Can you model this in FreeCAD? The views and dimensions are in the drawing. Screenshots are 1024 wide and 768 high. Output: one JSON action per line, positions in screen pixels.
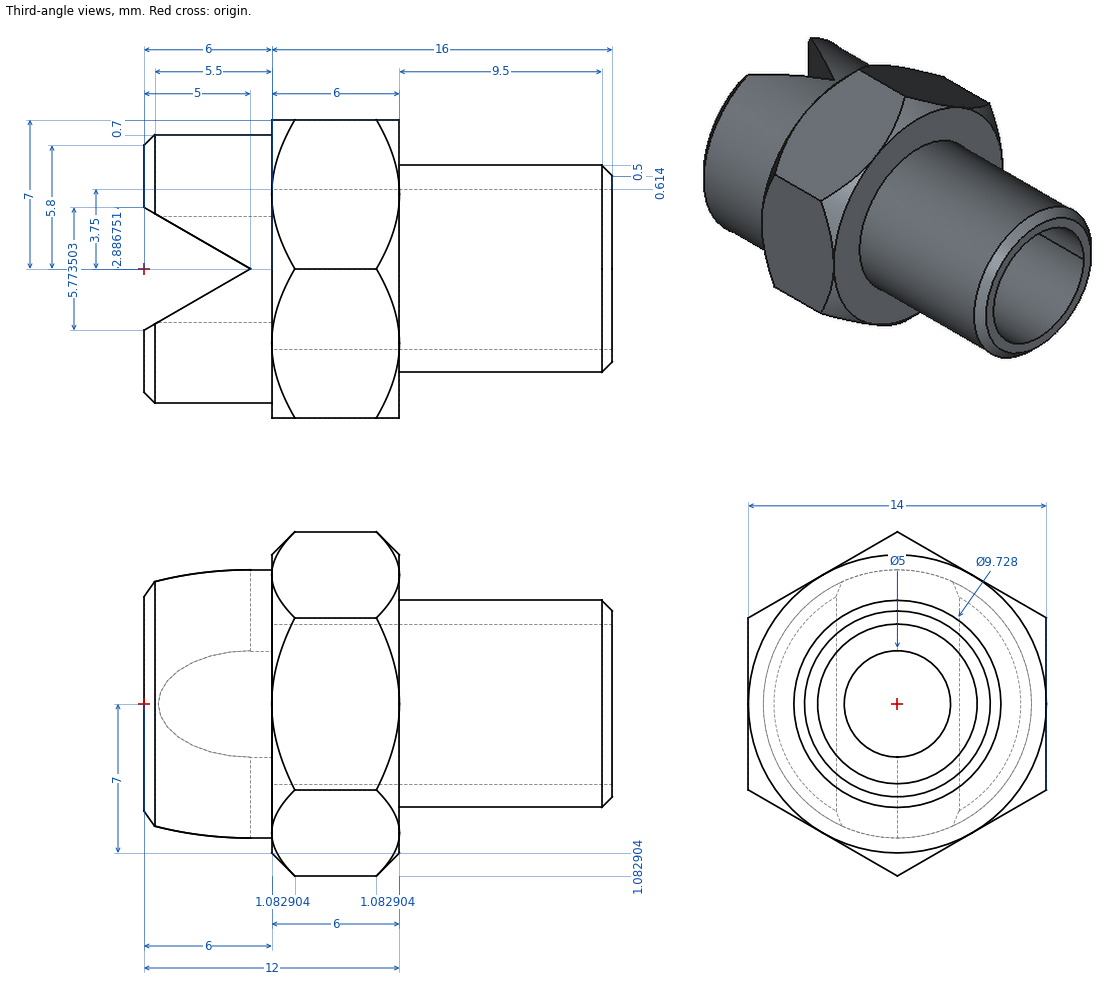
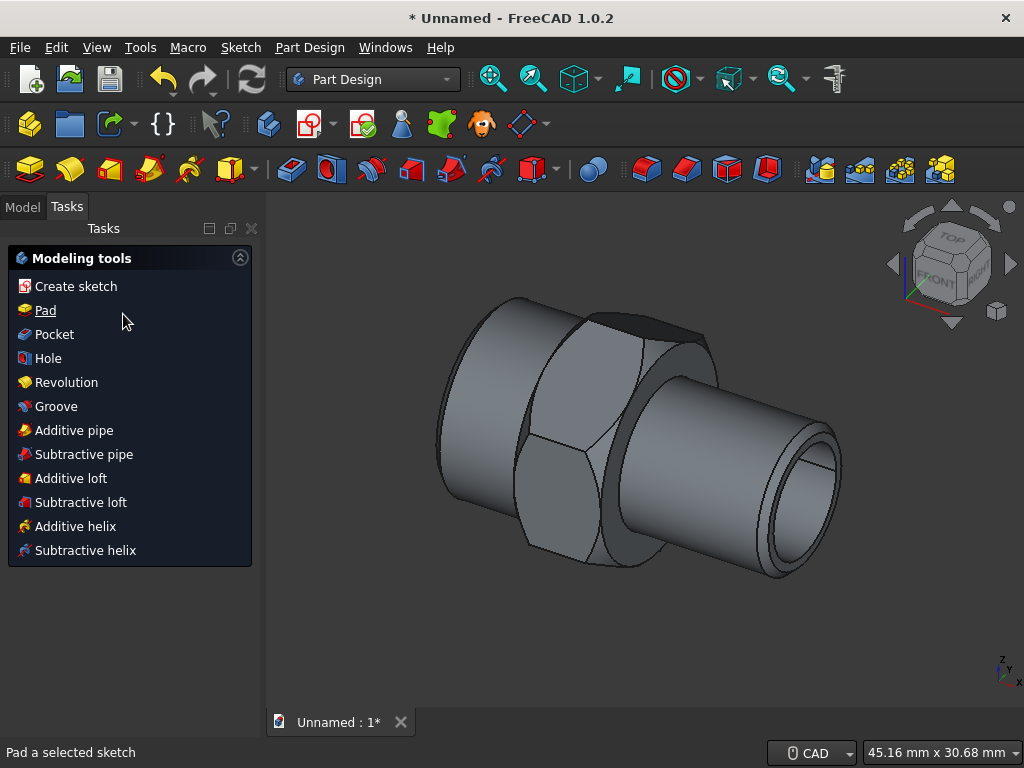
{"action": "left_click", "coordinate": [292, 170]}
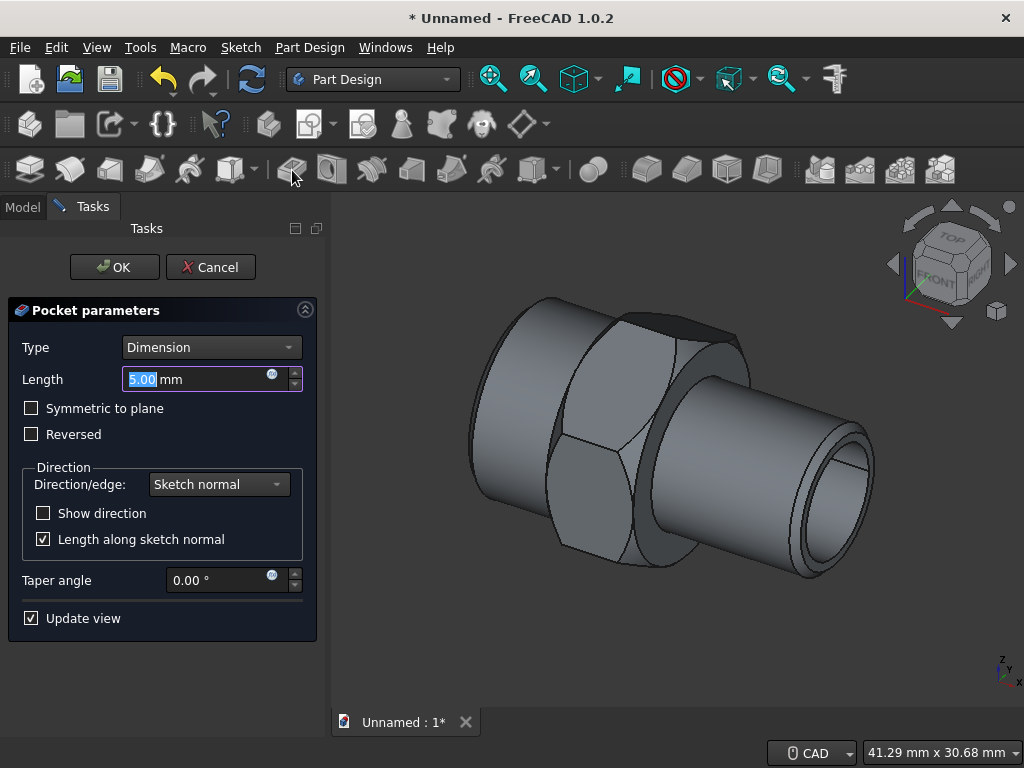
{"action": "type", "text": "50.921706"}
{"action": "key", "text": "Tab"}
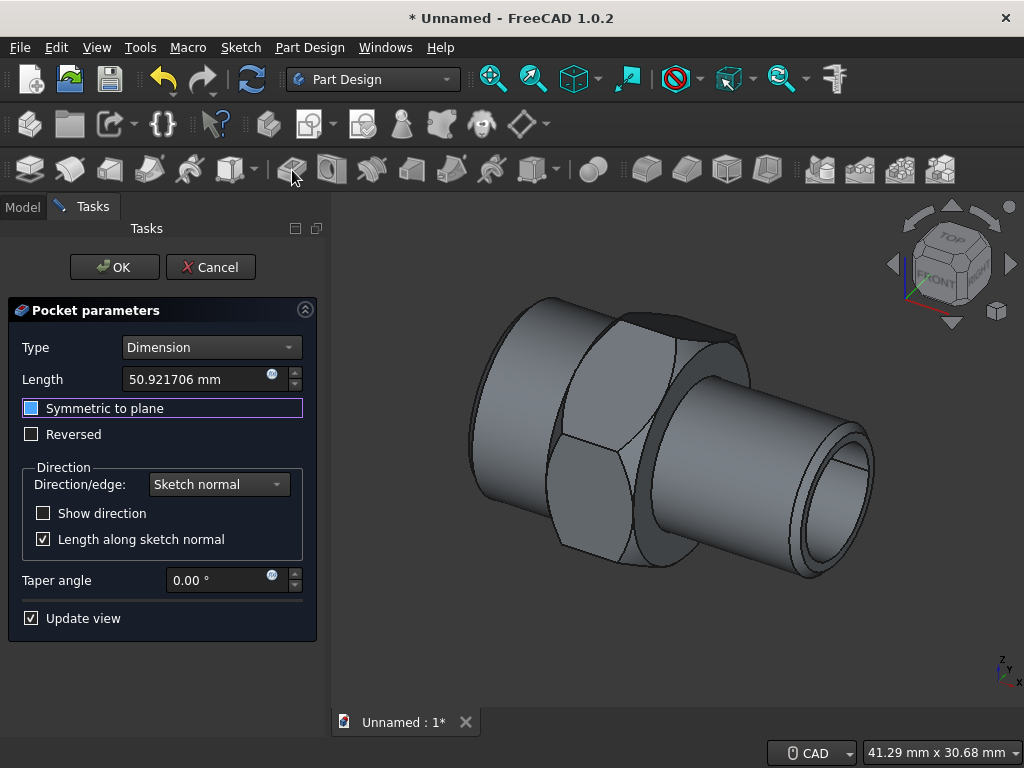
{"action": "left_click", "coordinate": [30, 408]}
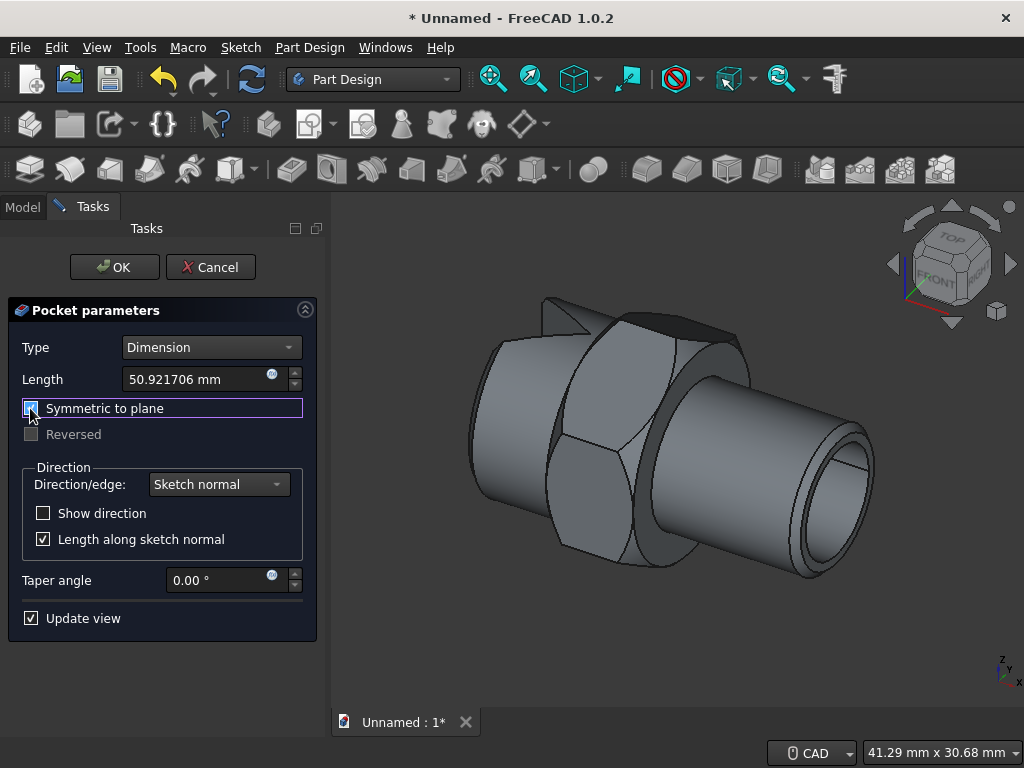
{"action": "left_click", "coordinate": [115, 267]}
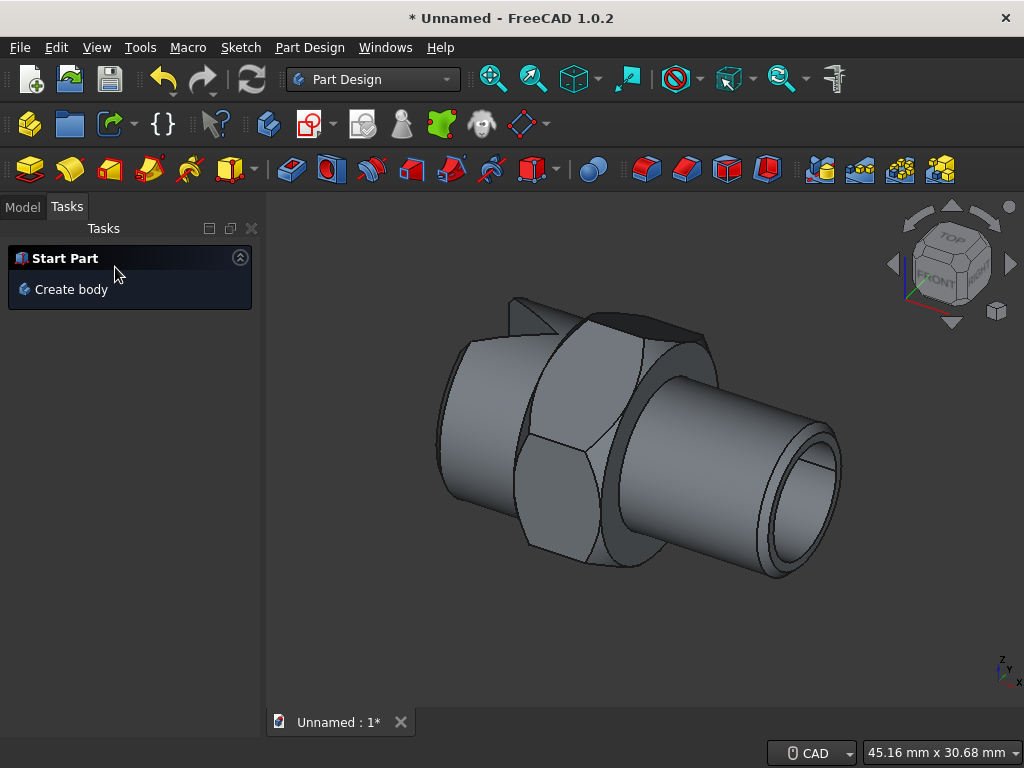
{"action": "key", "text": "0"}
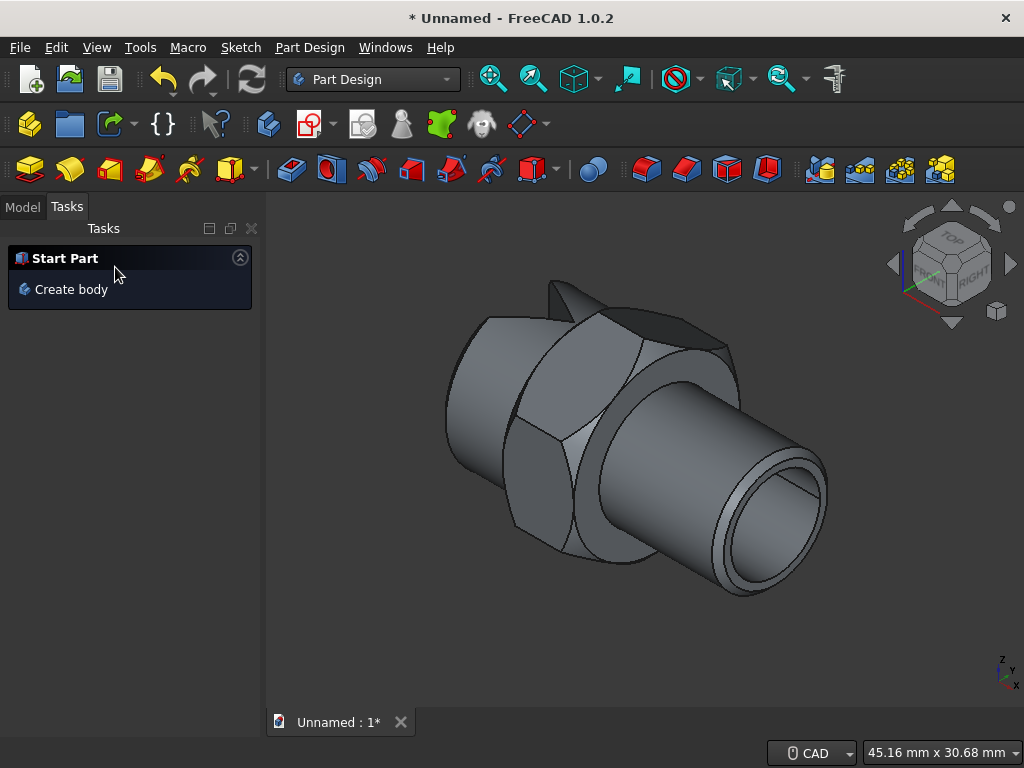
{"action": "key", "text": "3"}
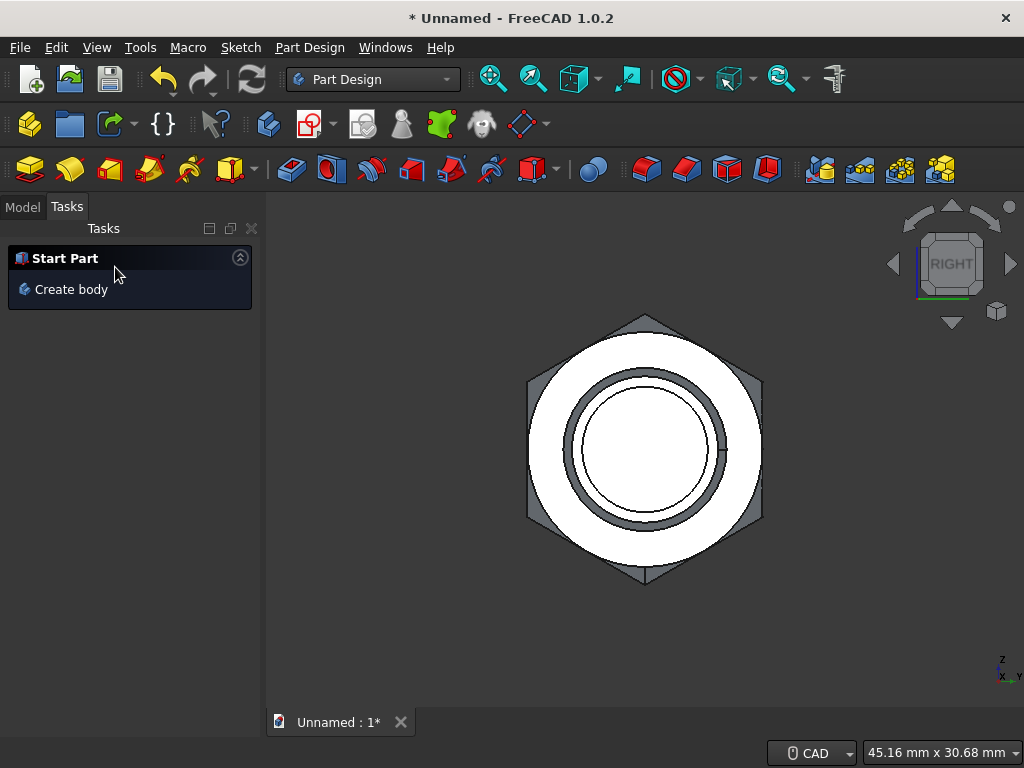
{"action": "left_click", "coordinate": [645, 448]}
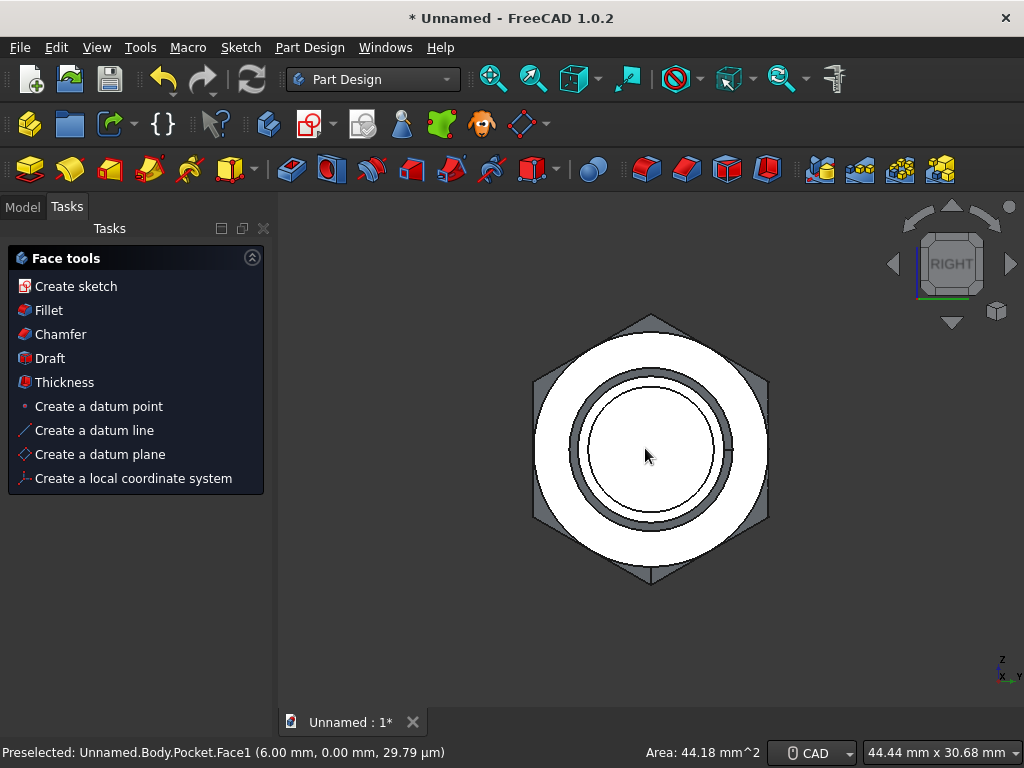
{"action": "left_click", "coordinate": [310, 124]}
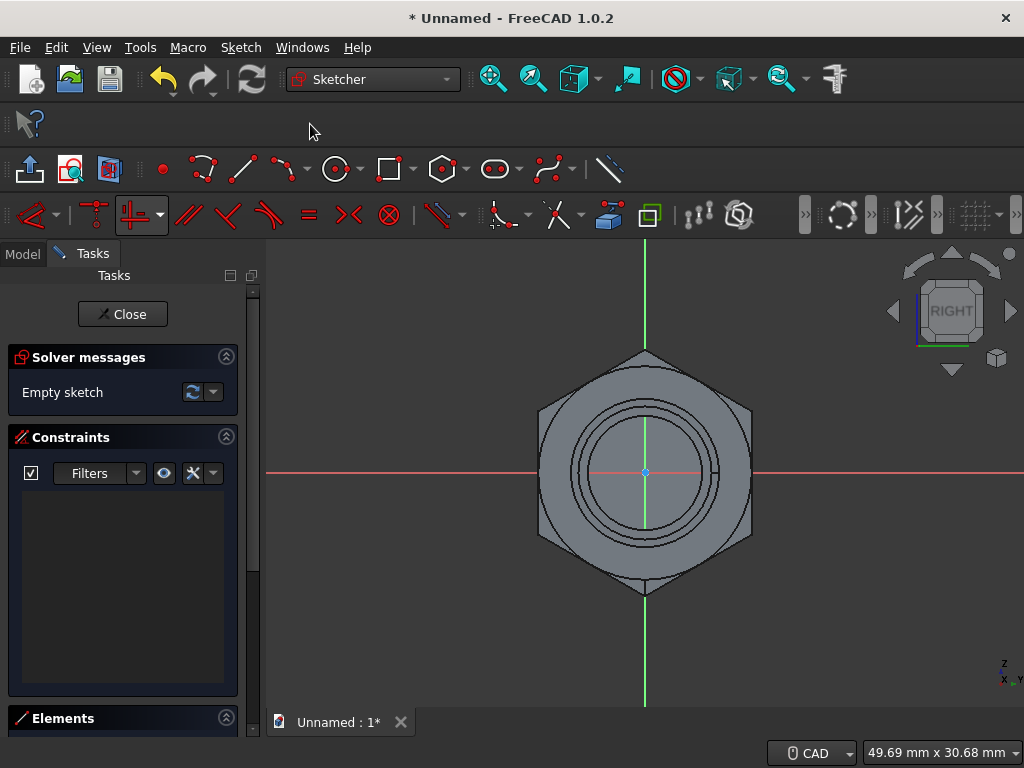
{"action": "scroll", "coordinate": [667, 473], "scroll_direction": "up", "scroll_amount": 7}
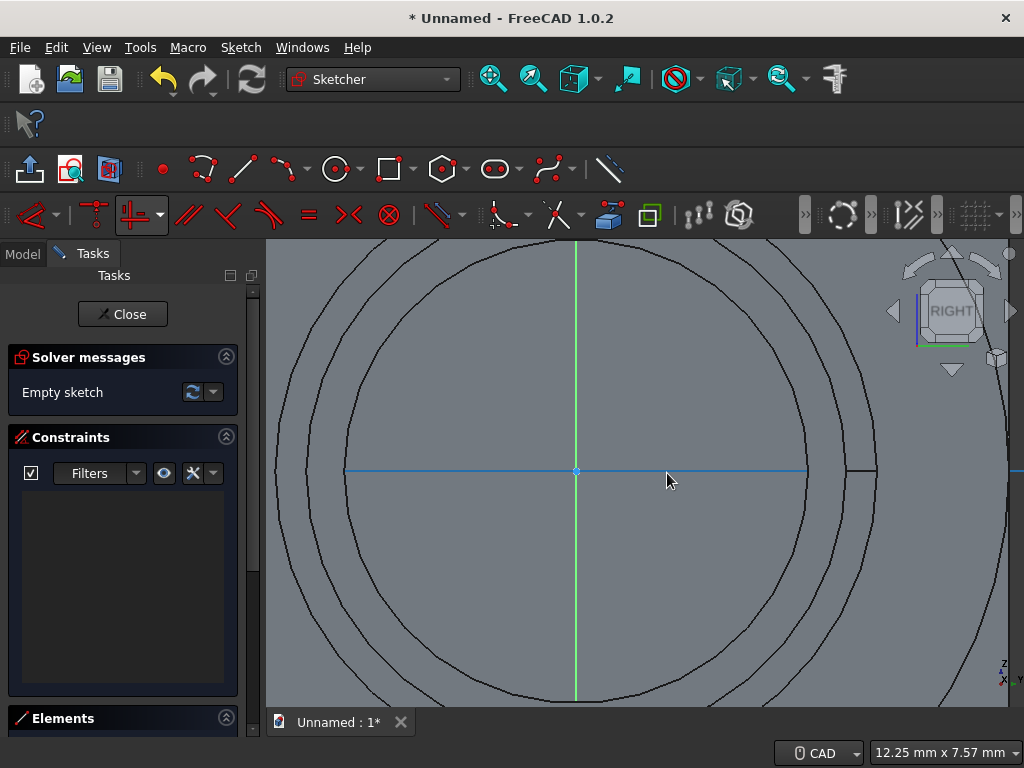
{"action": "left_click", "coordinate": [336, 170]}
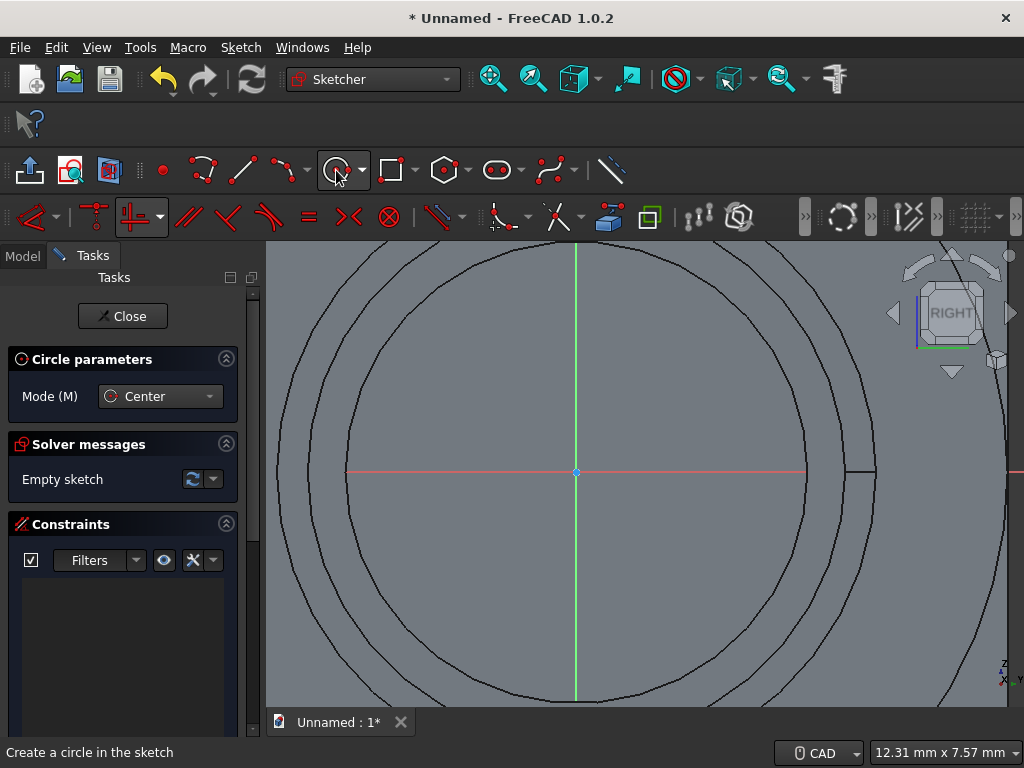
{"action": "left_click", "coordinate": [576, 472]}
{"action": "left_click", "coordinate": [685, 364]}
{"action": "key", "text": "Escape"}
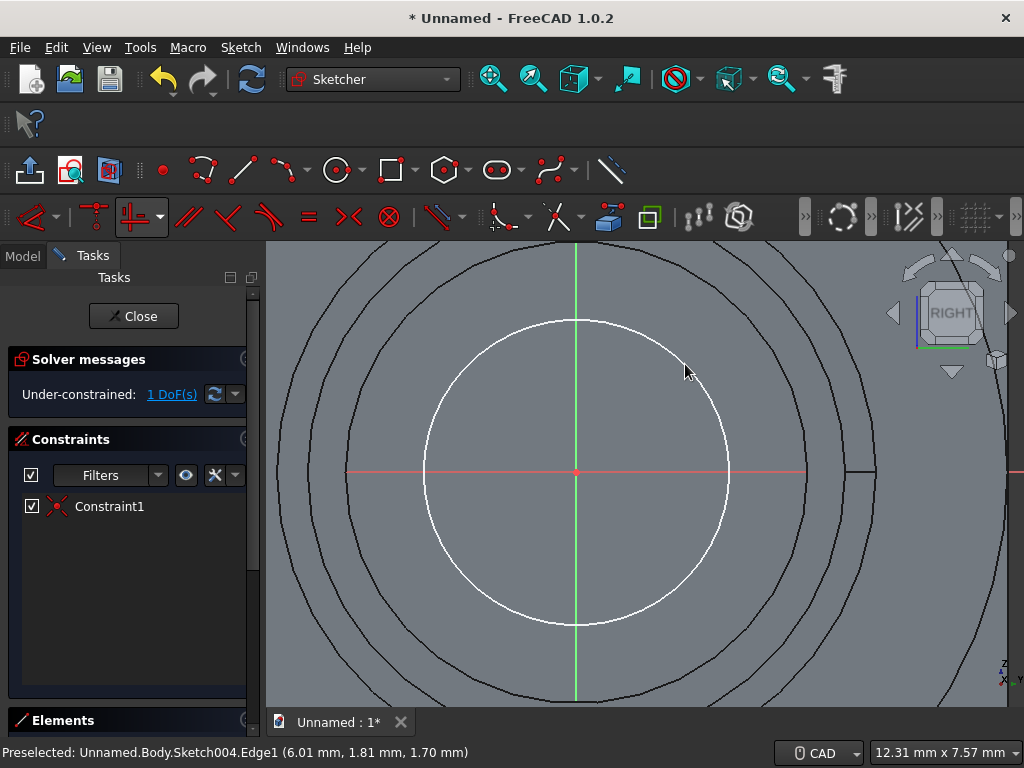
{"action": "left_click", "coordinate": [32, 218]}